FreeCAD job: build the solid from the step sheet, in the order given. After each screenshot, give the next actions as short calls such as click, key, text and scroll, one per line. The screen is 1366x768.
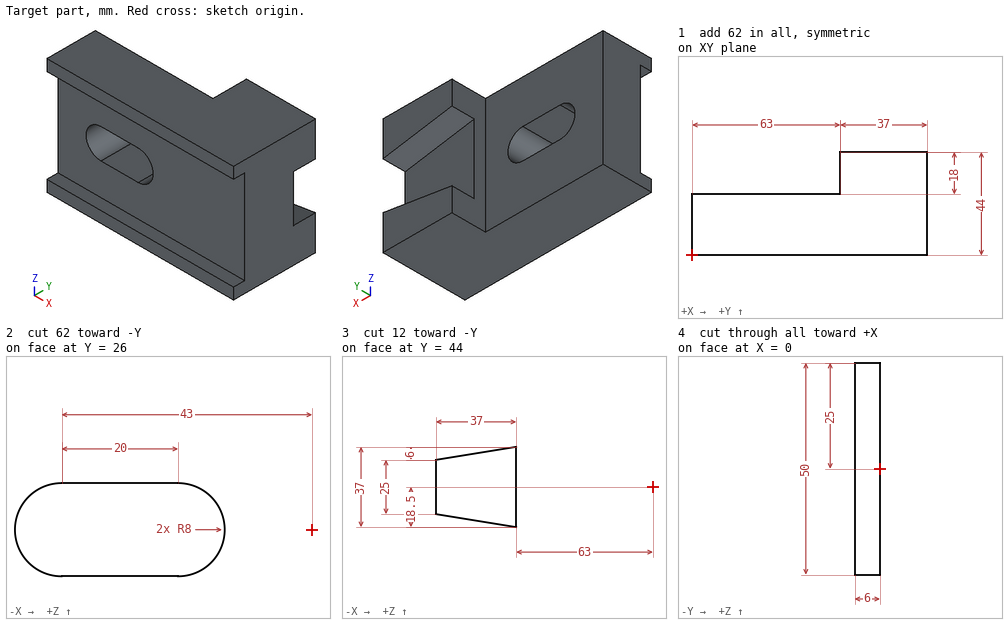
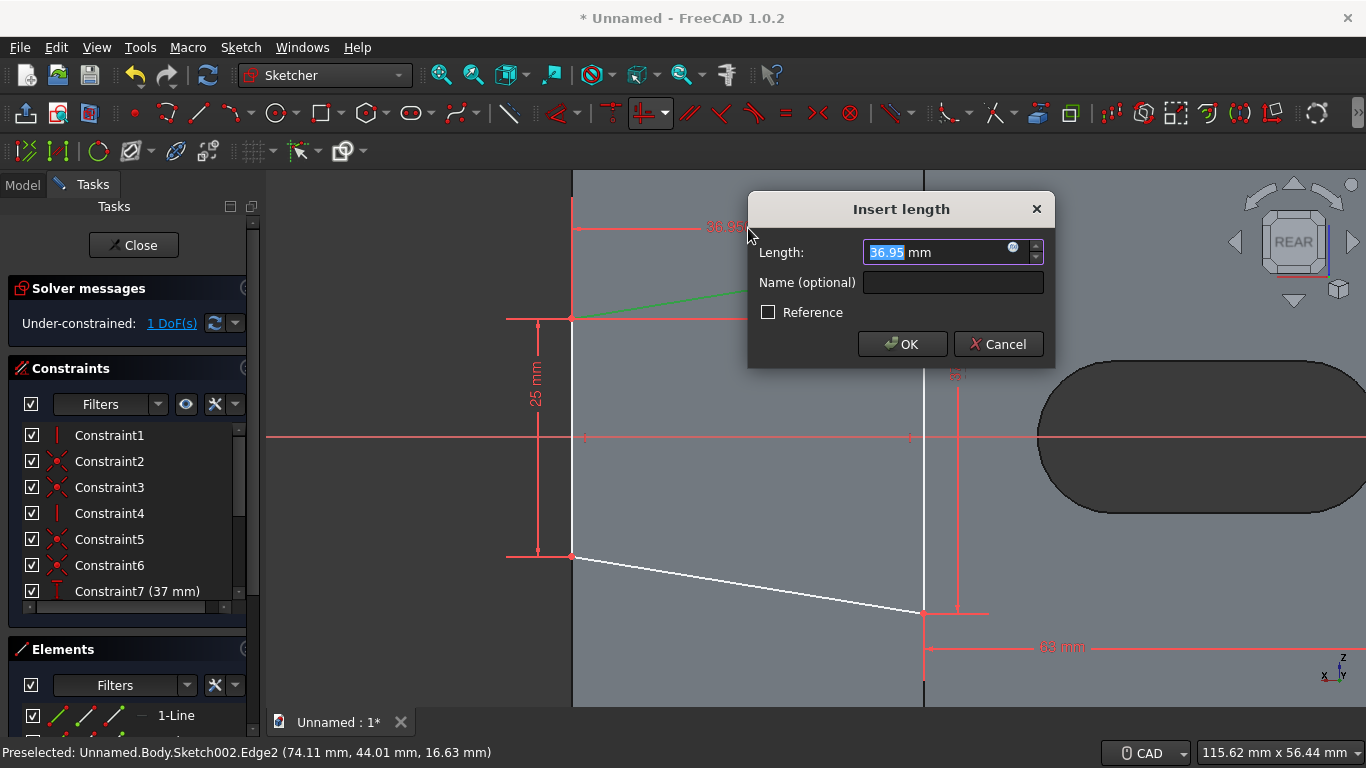
text(37)
key(Return)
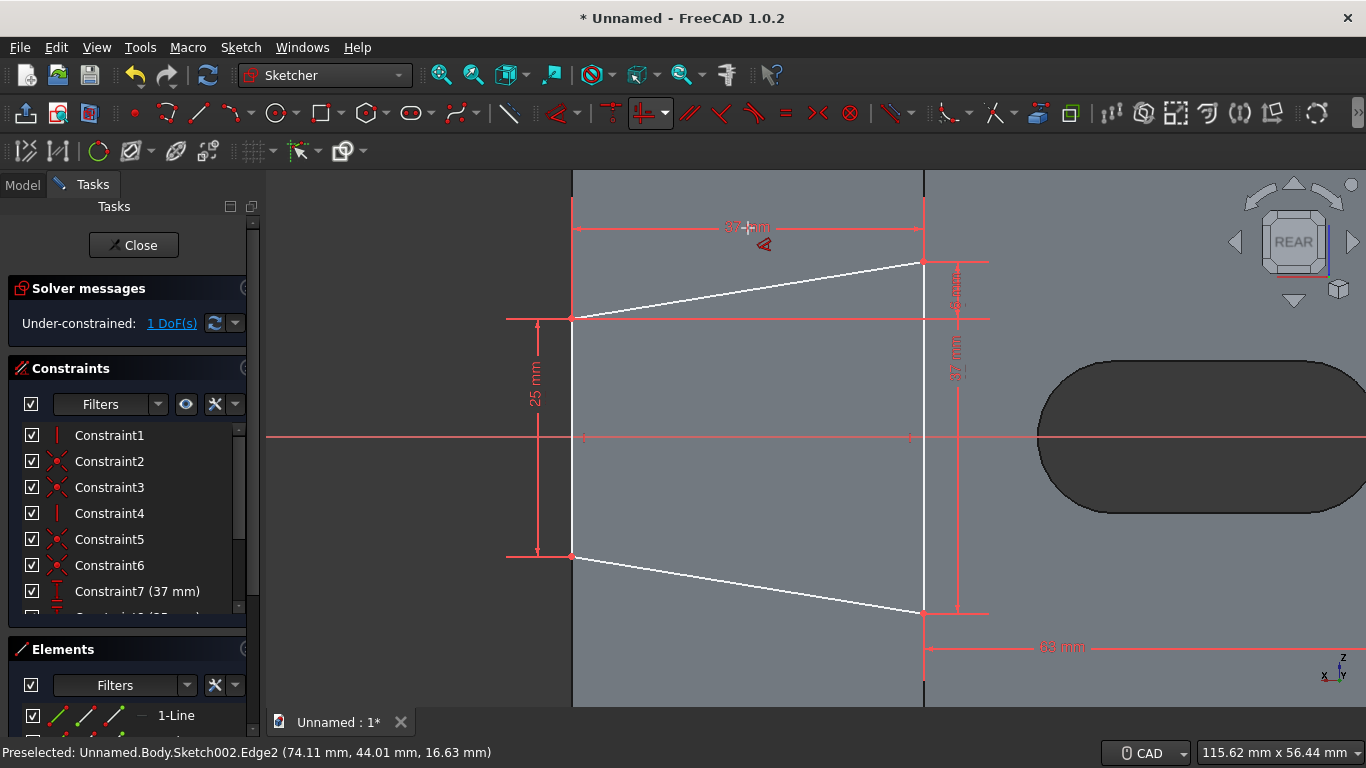
click(924, 614)
click(890, 526)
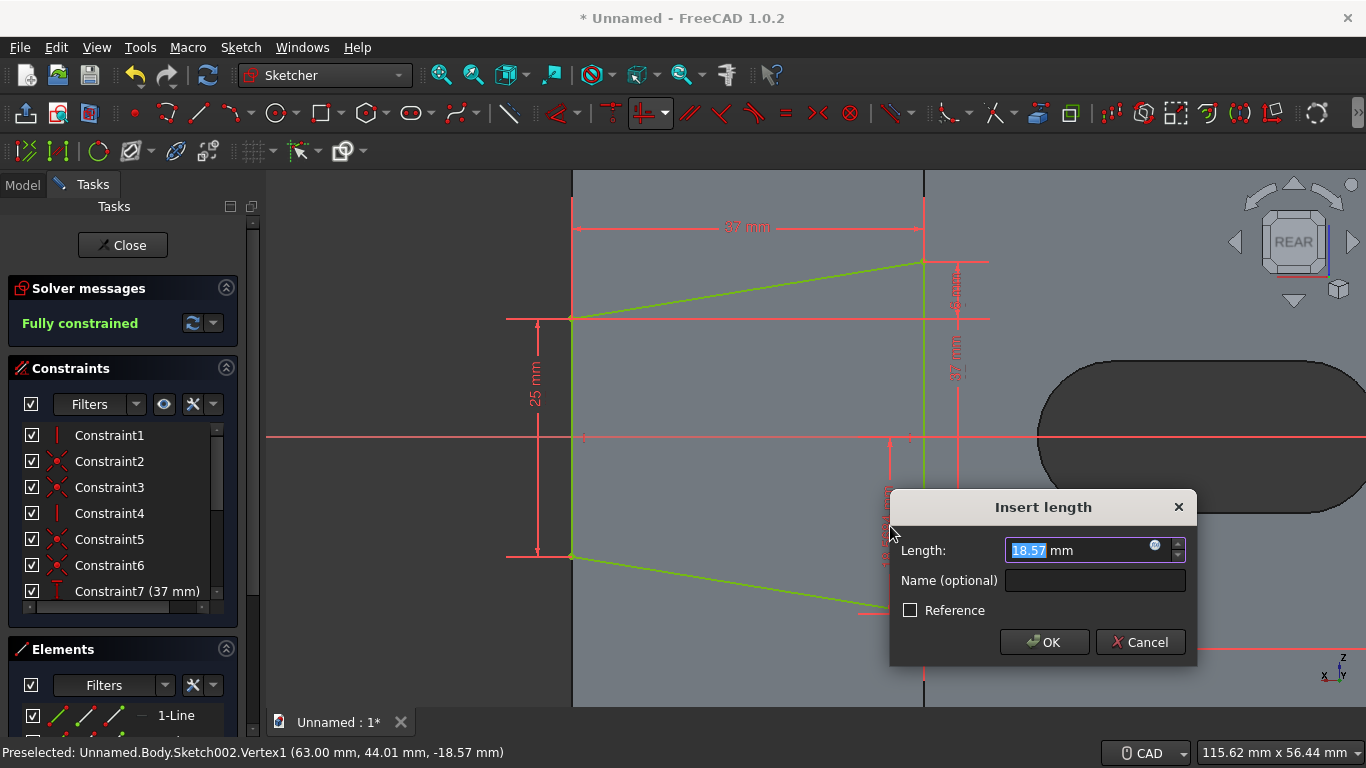
text(18.5)
key(Return)
key(Escape)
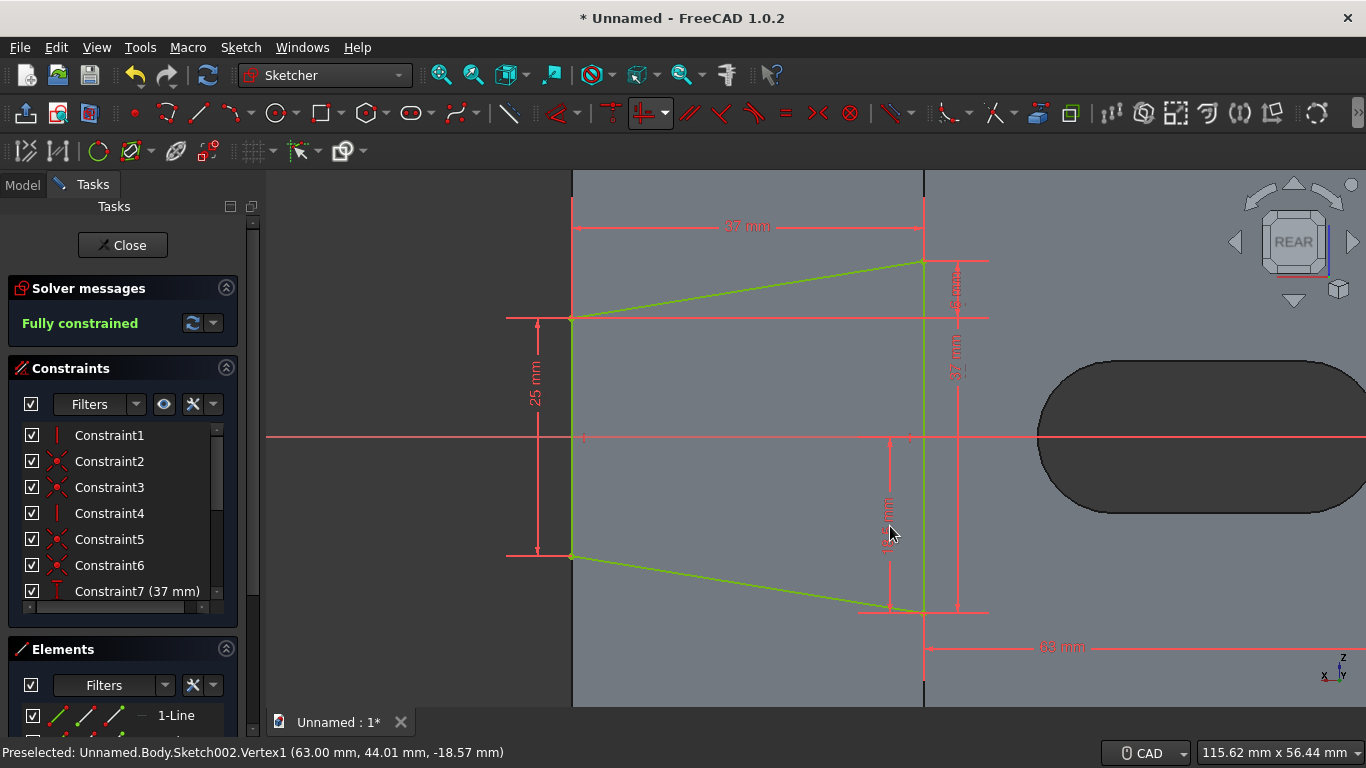
click(123, 245)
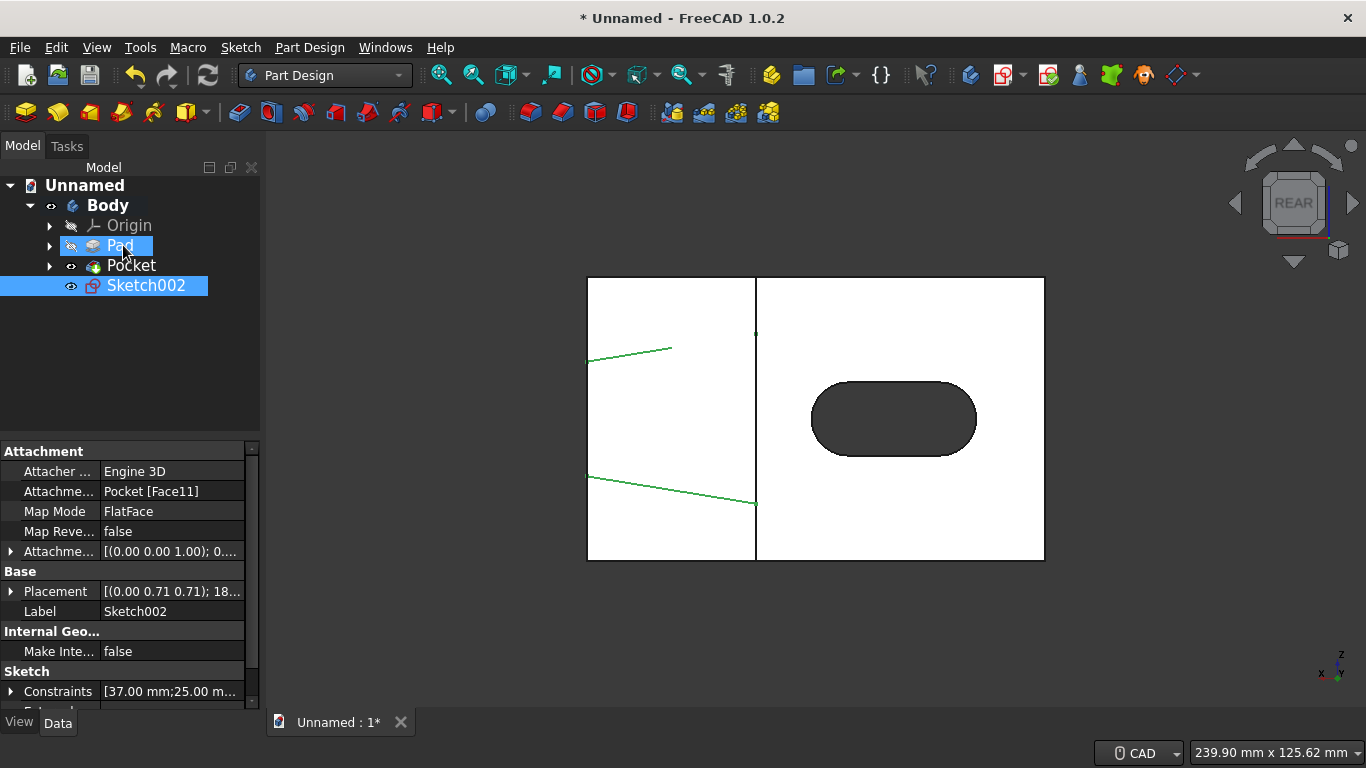
click(240, 112)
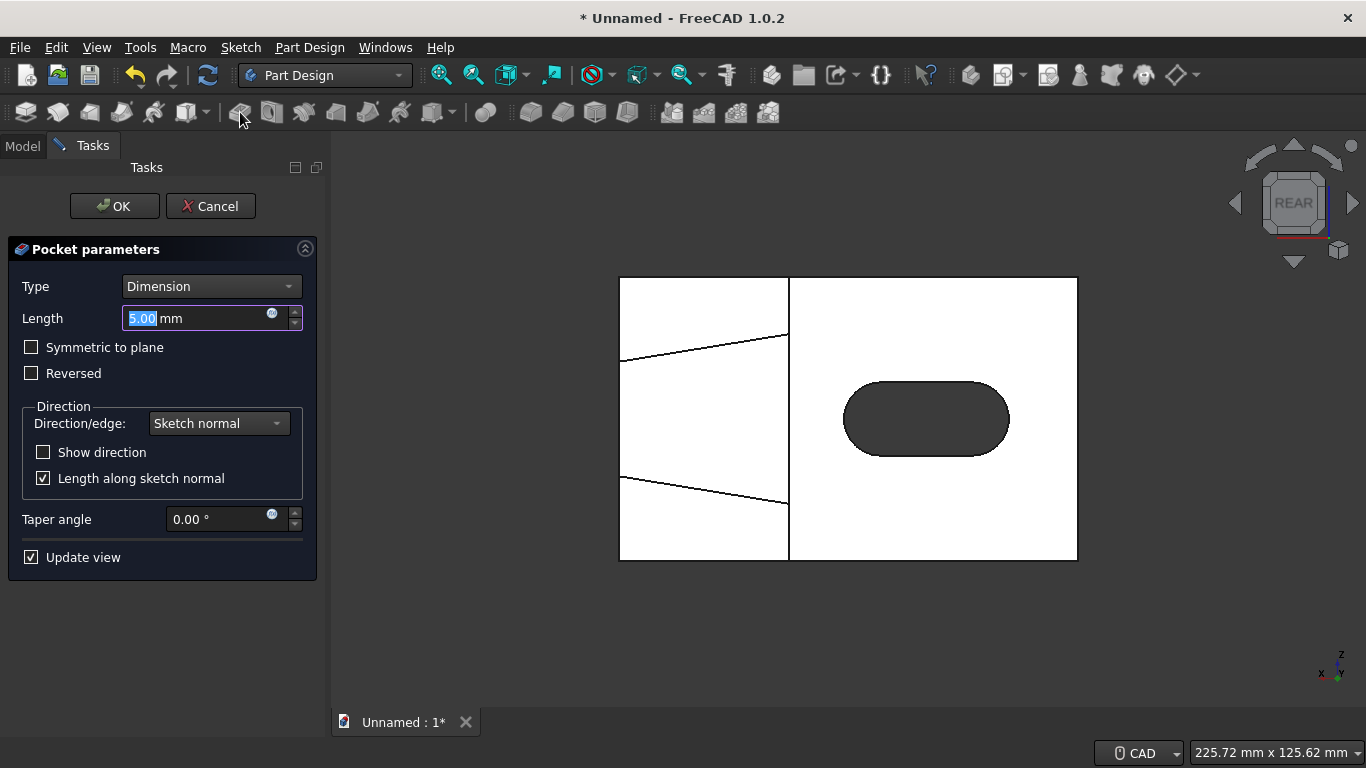
text(12)
key(Tab)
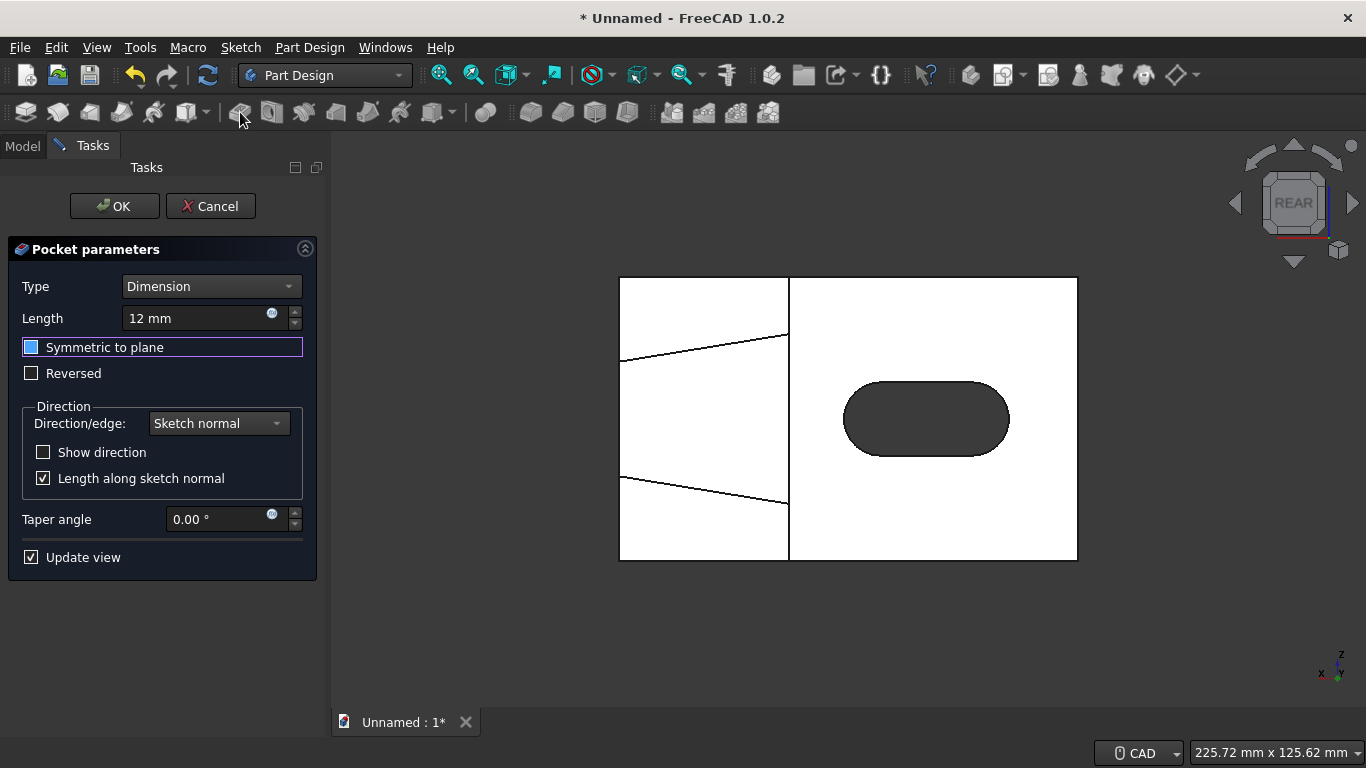
click(115, 206)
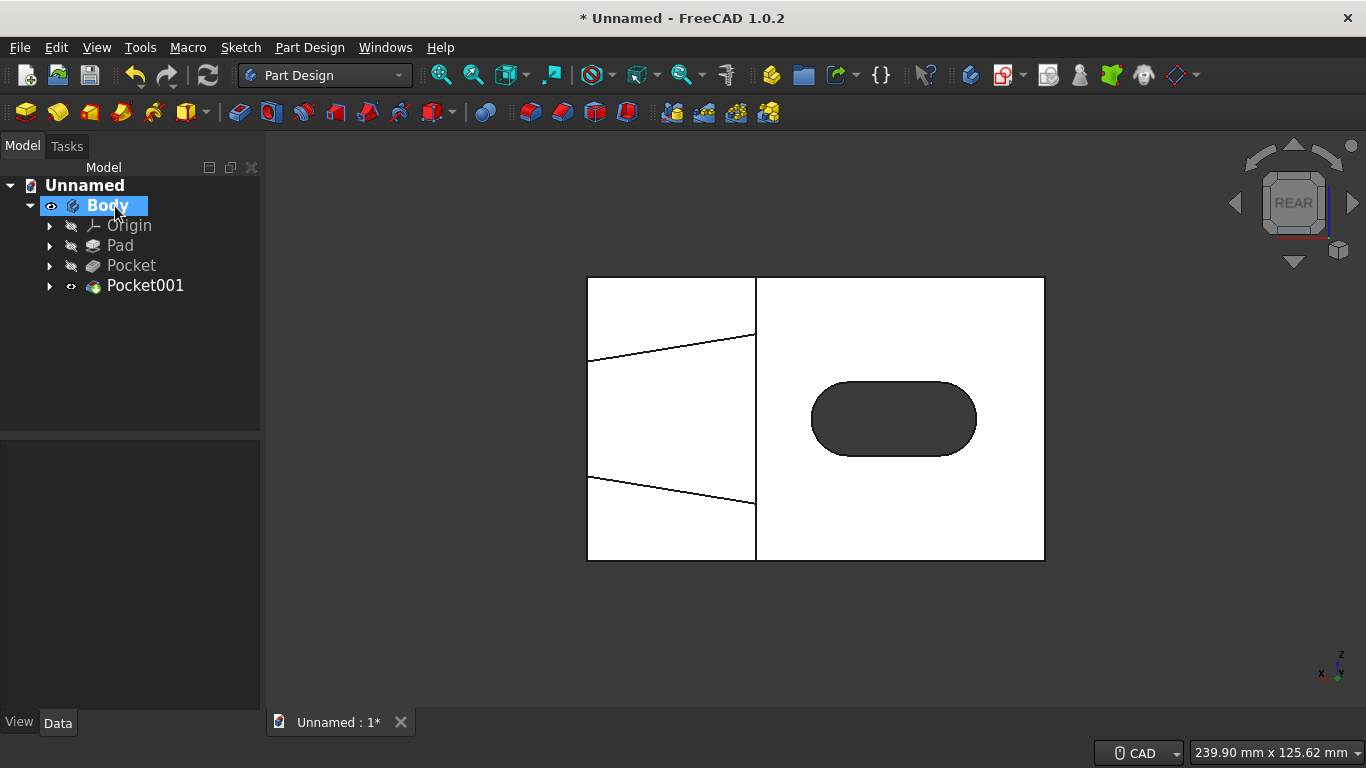
key(6)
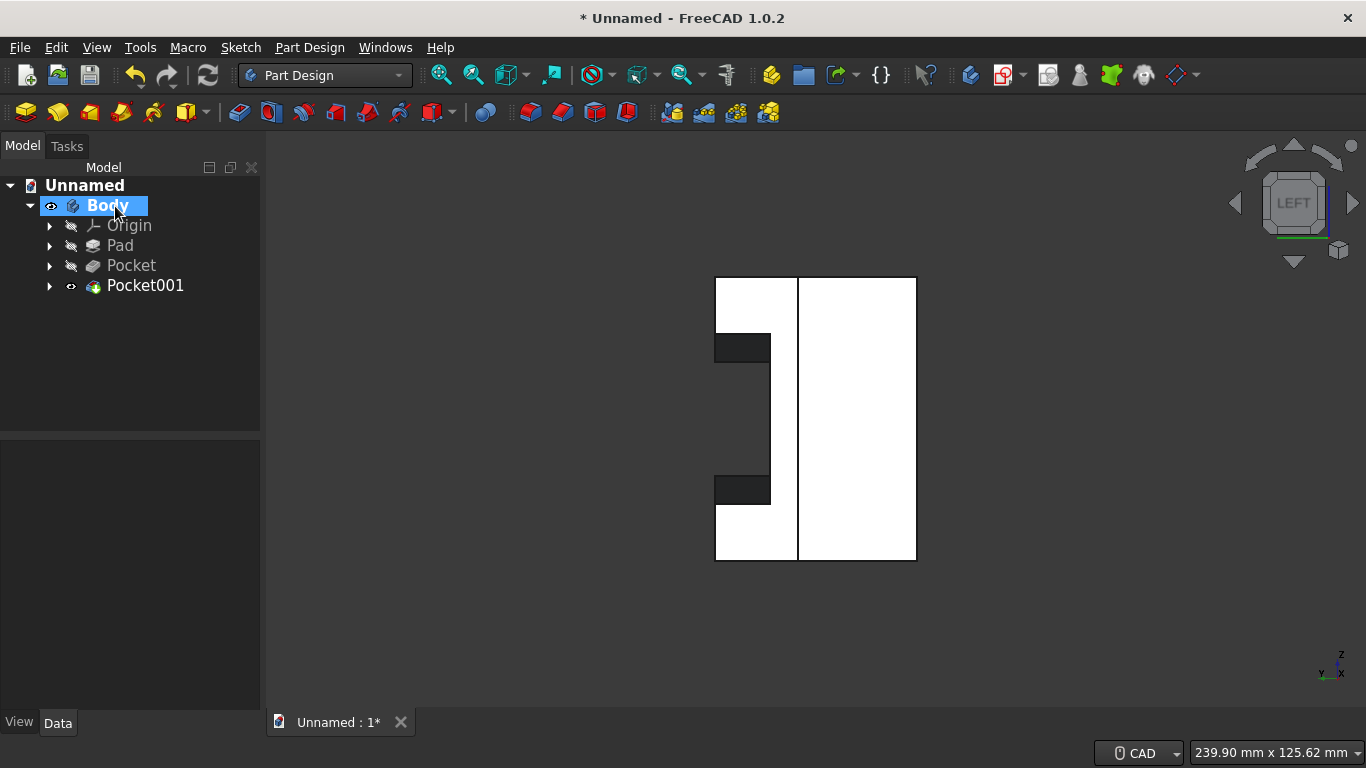
click(857, 337)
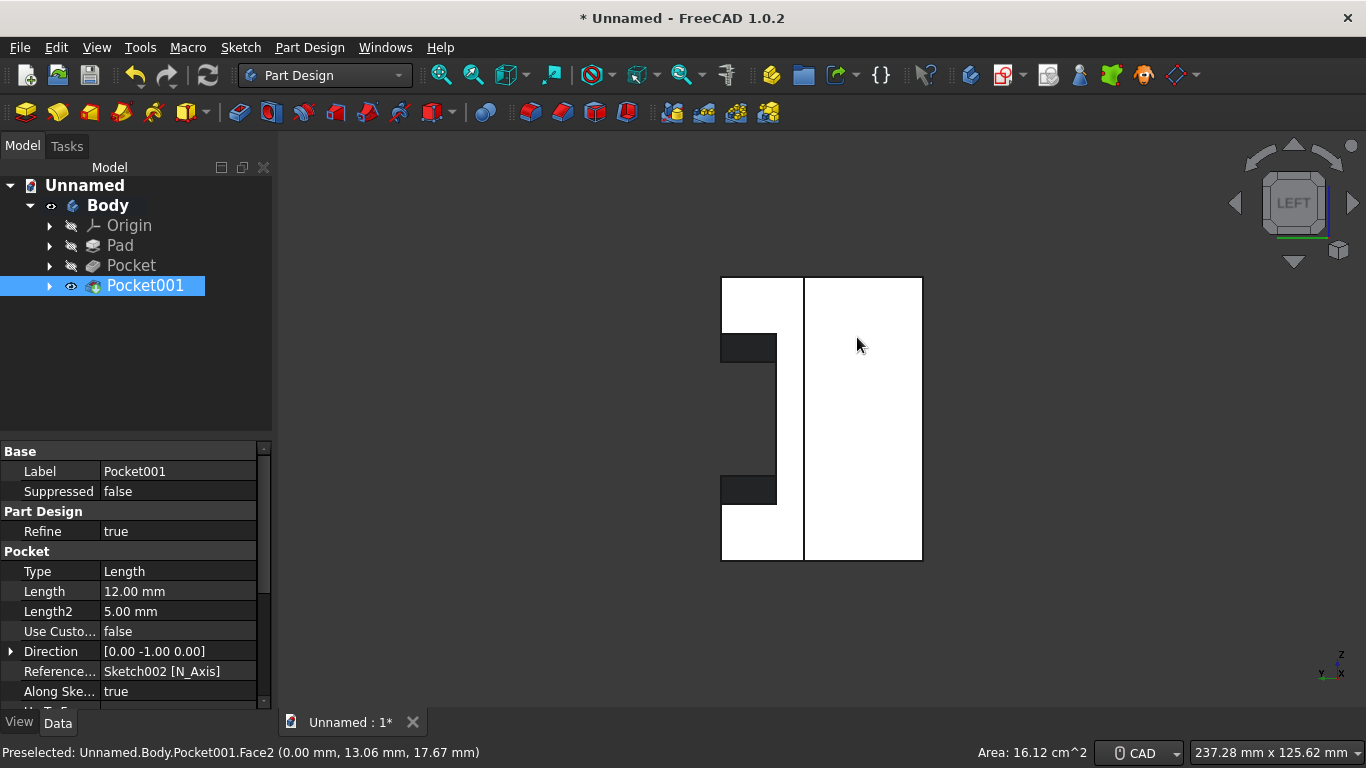
click(1004, 76)